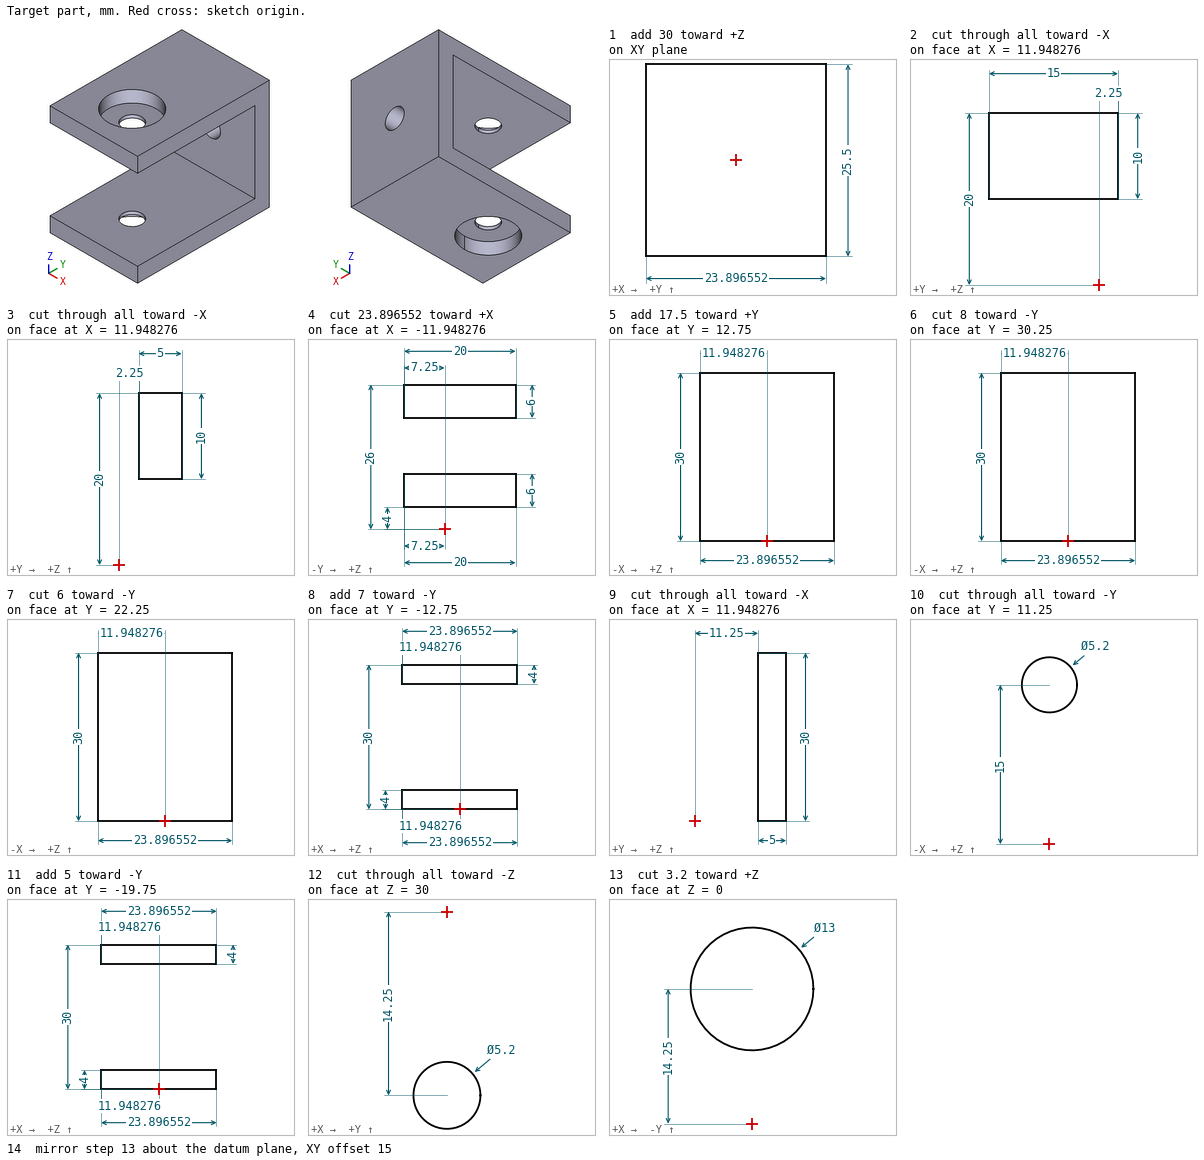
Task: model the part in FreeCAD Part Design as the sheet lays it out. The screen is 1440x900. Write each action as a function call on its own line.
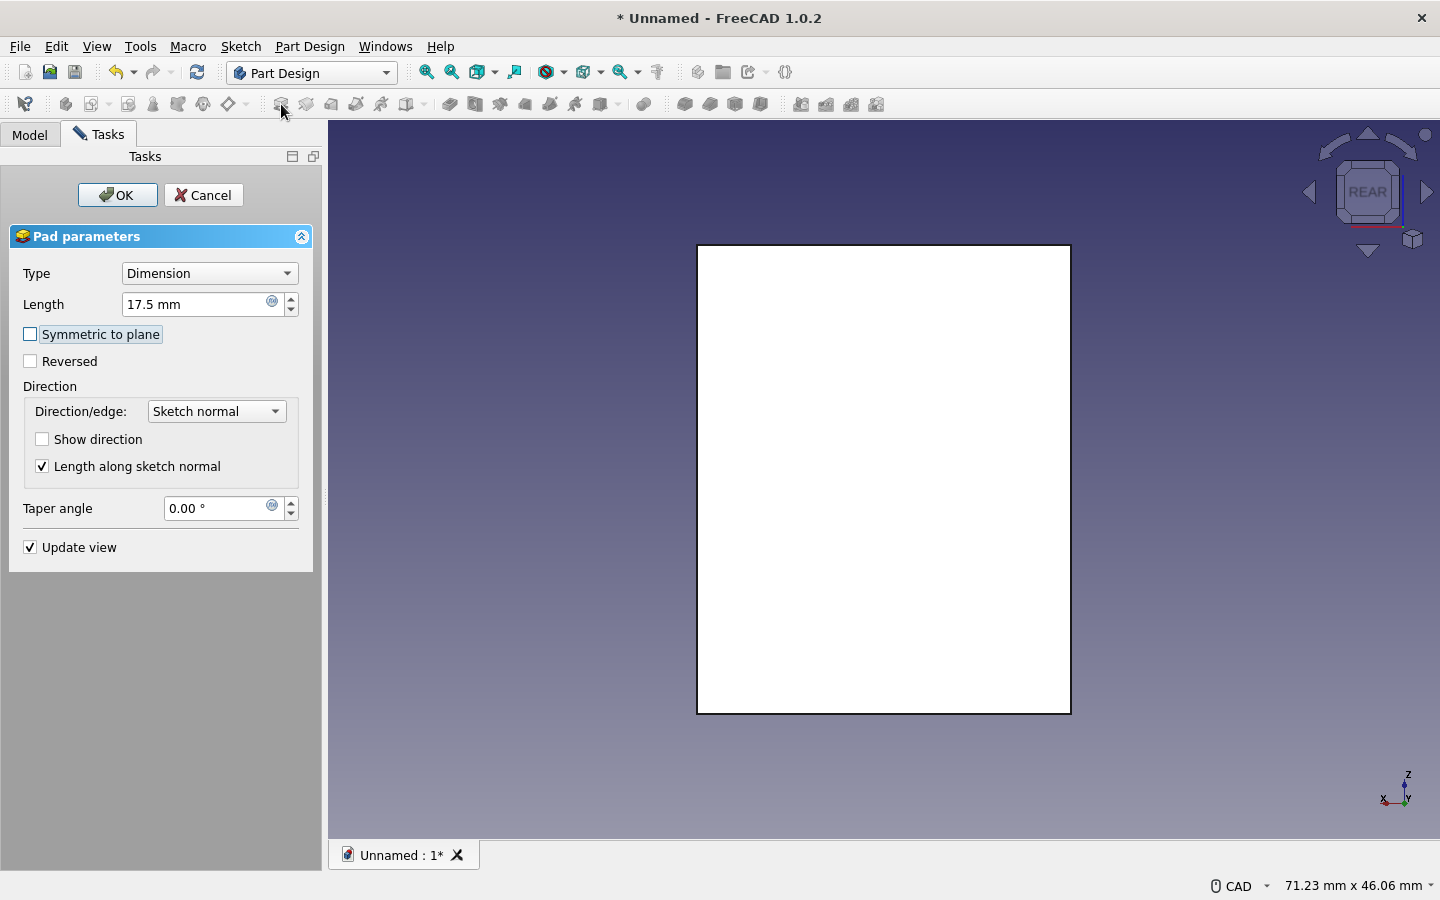
click(118, 195)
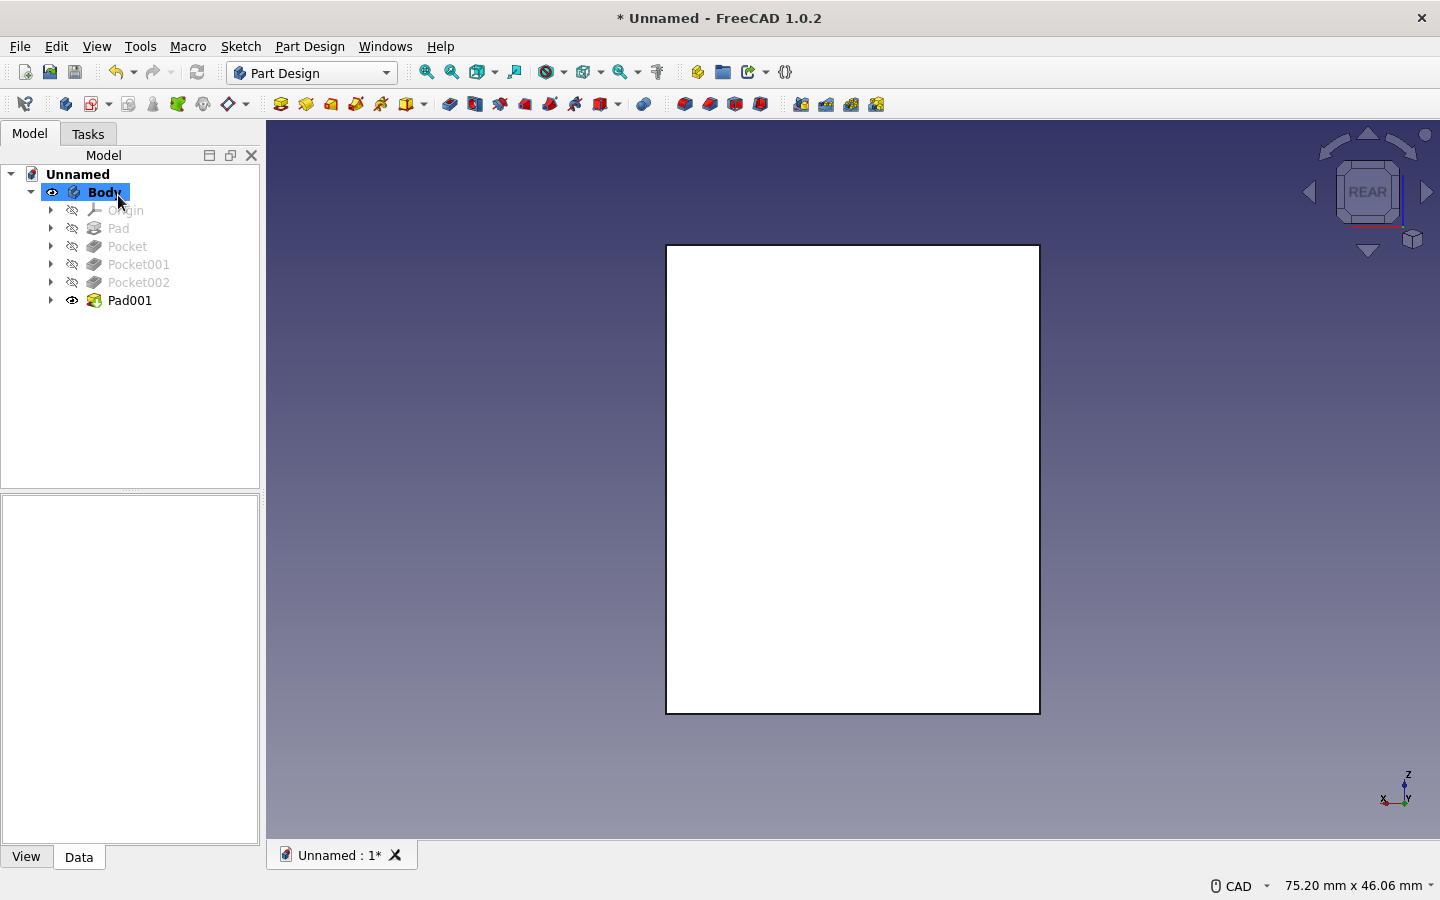
click(853, 479)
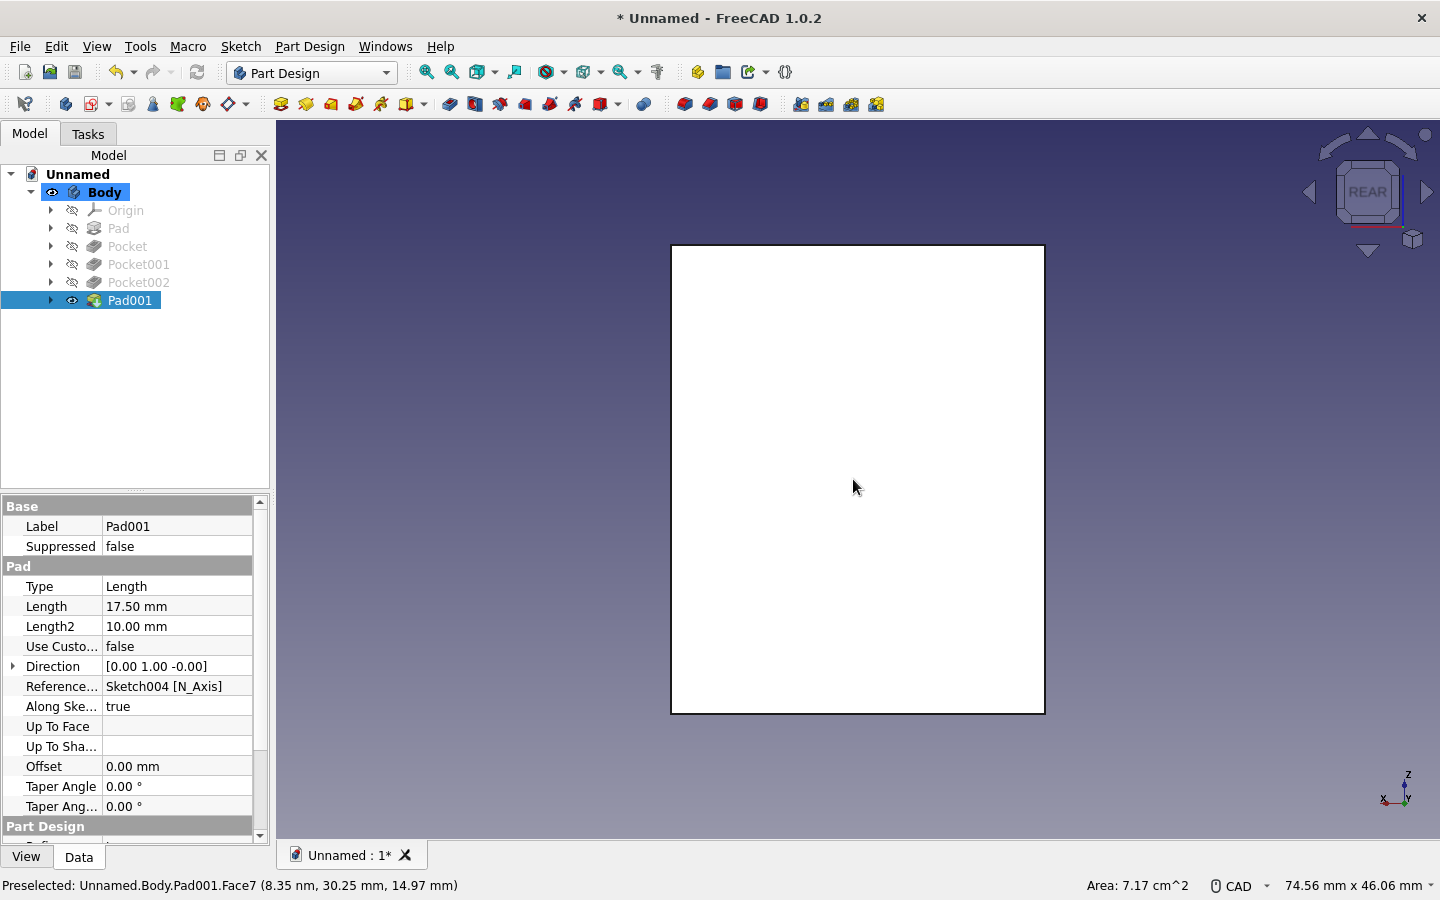
click(90, 104)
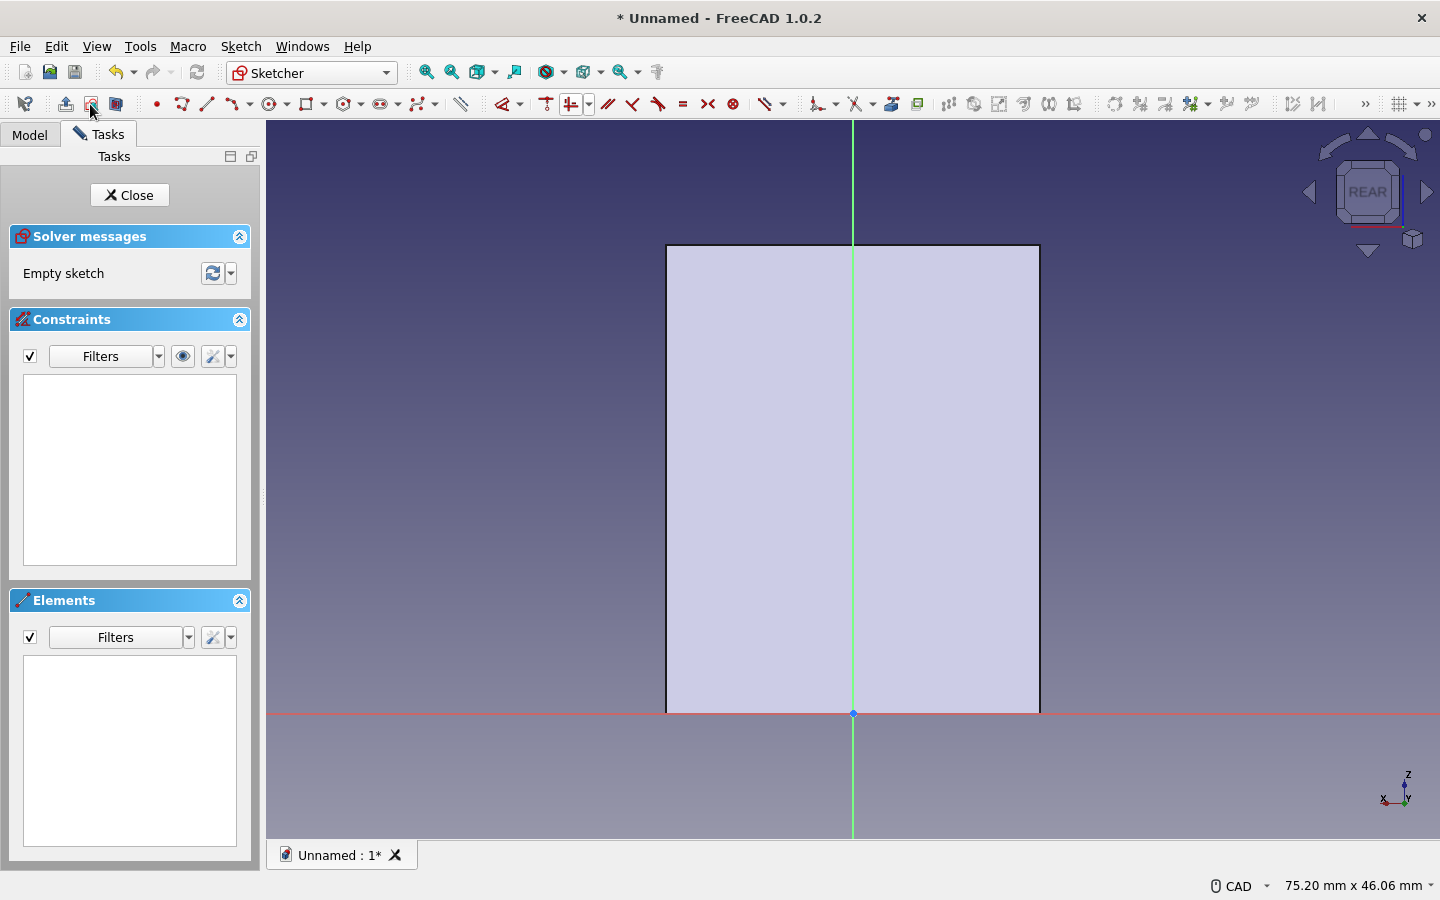
click(306, 104)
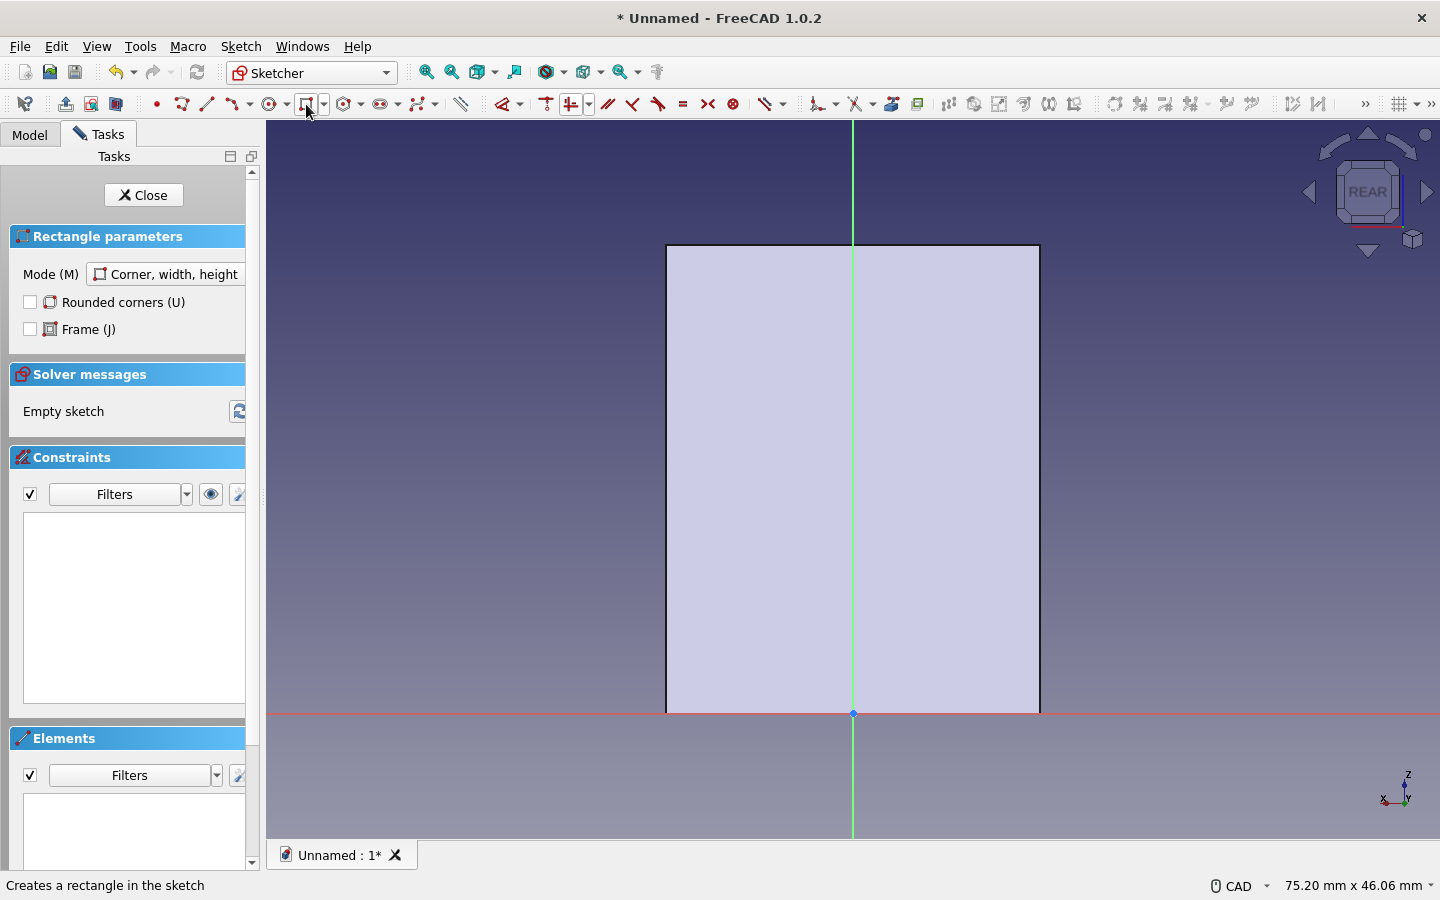
click(666, 245)
click(1040, 714)
key(Escape)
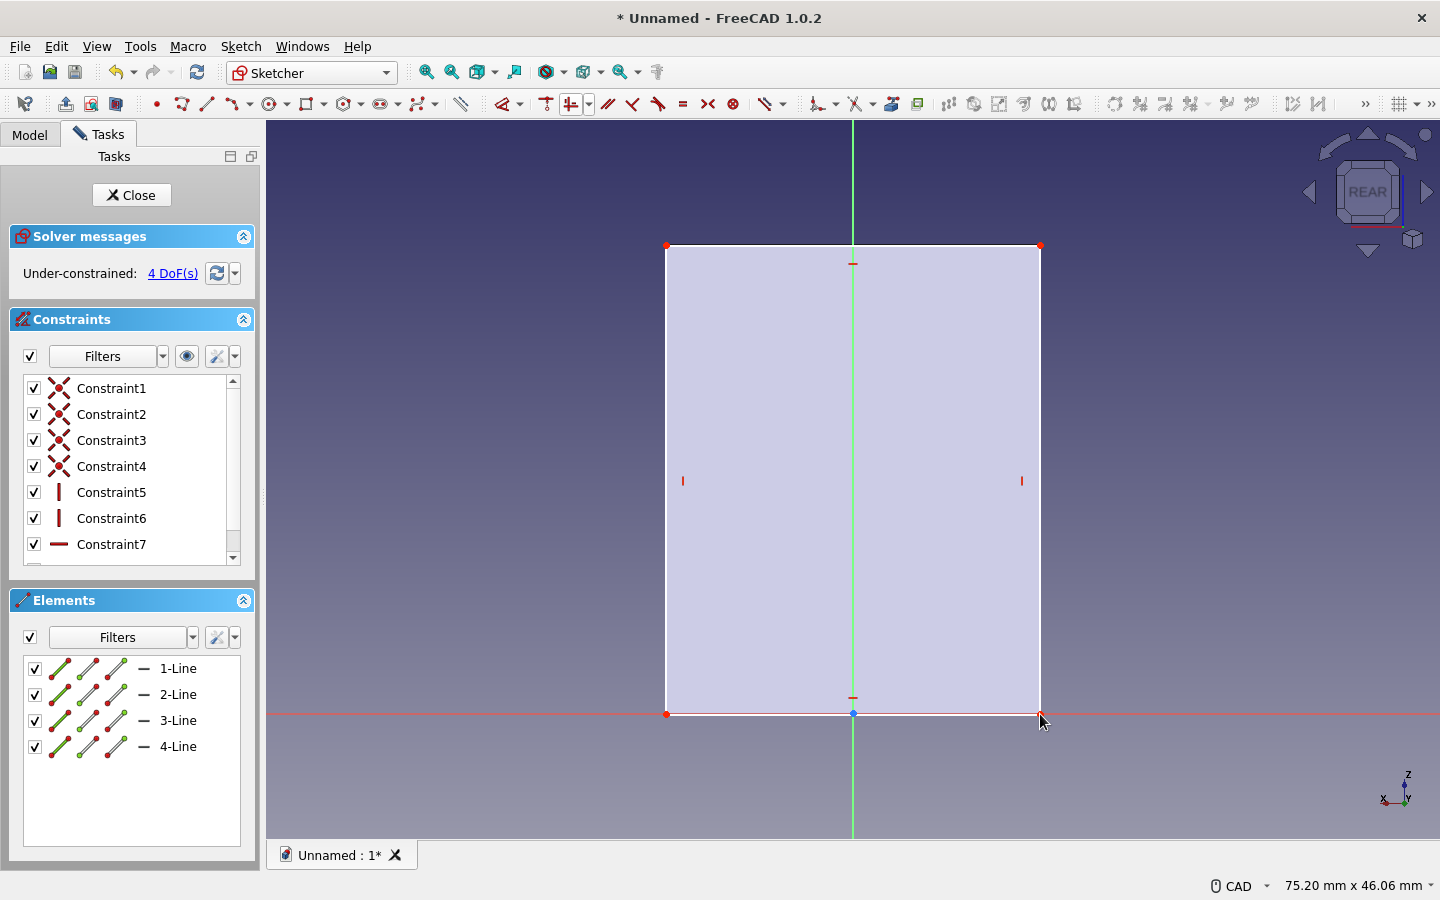
click(666, 715)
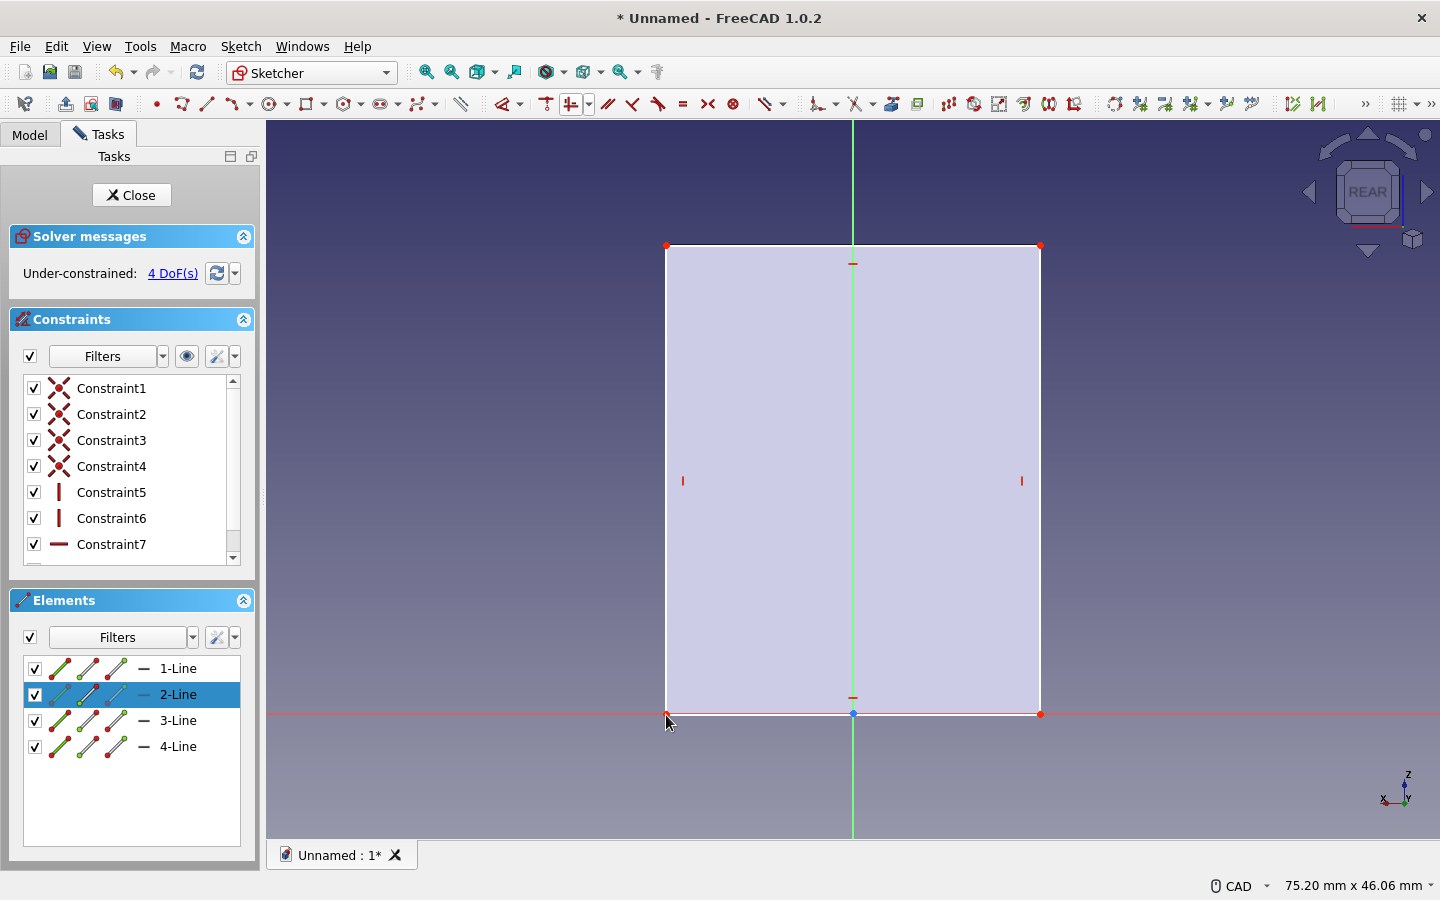
click(364, 714)